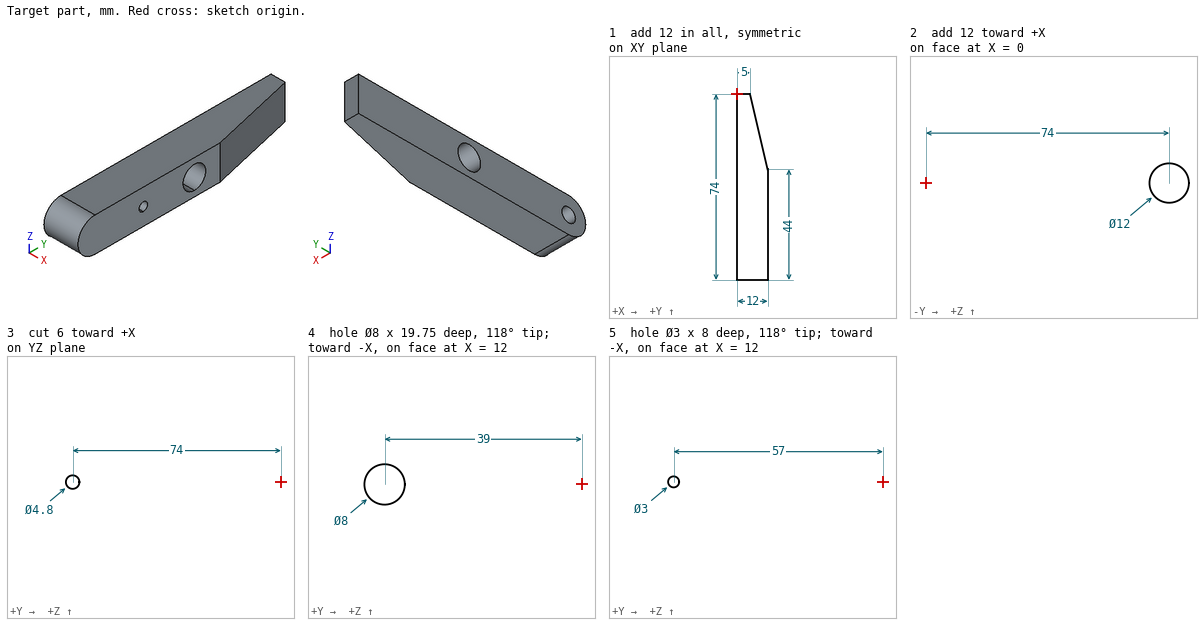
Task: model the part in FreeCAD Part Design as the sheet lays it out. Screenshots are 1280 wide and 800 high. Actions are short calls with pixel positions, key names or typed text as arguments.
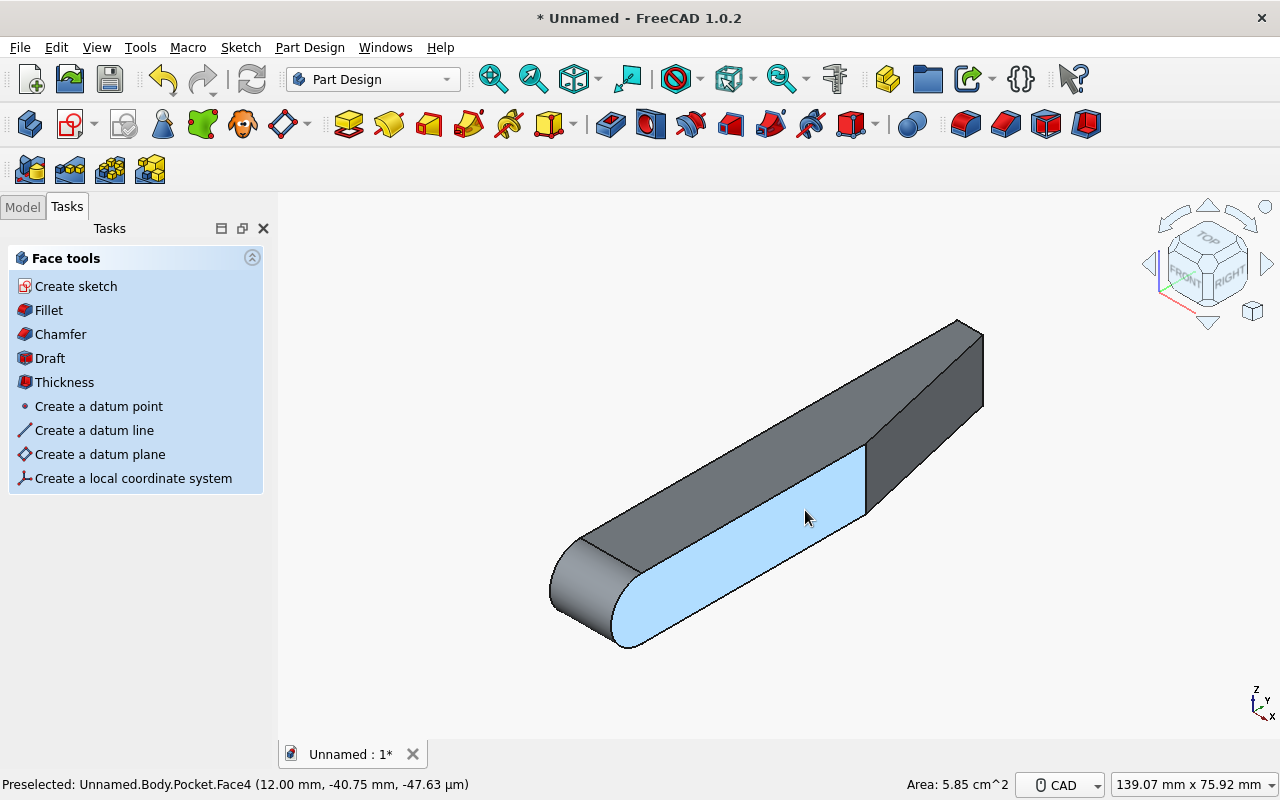
click(70, 124)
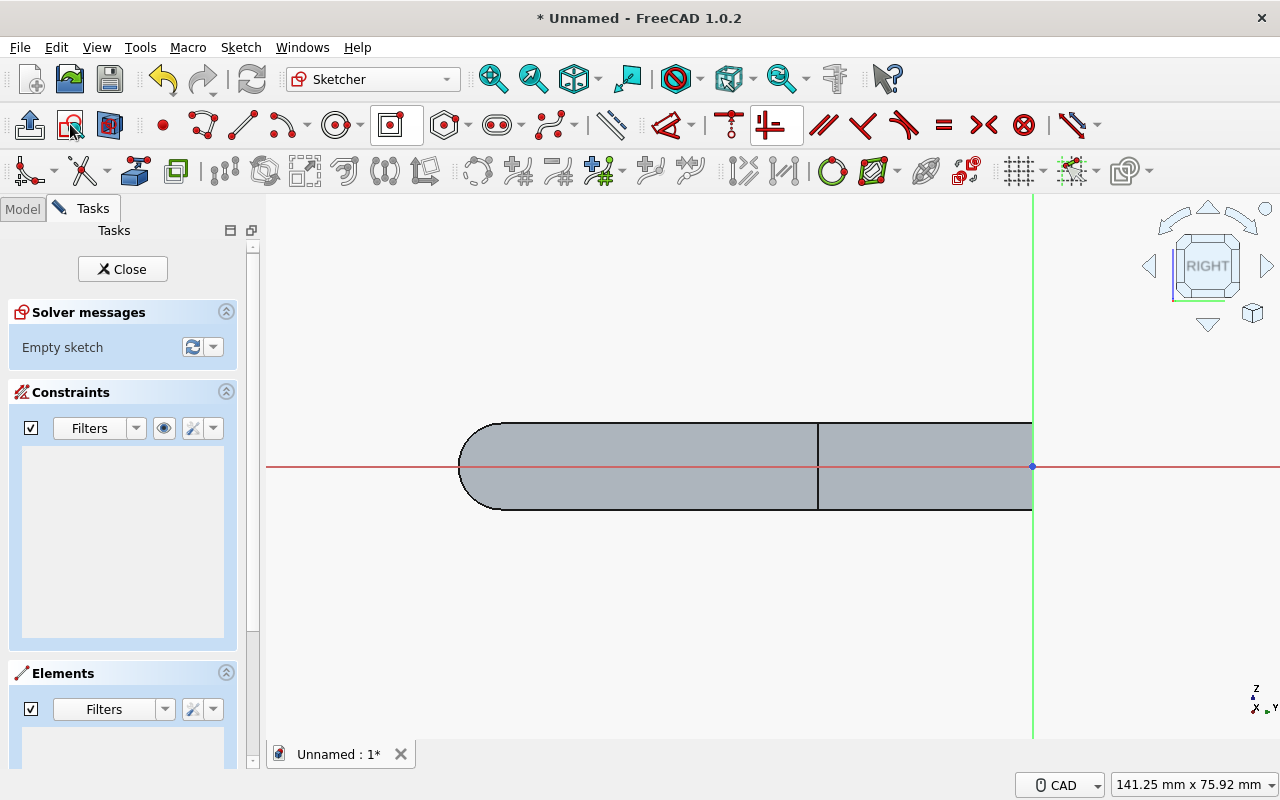
scroll(762, 467, up, 9)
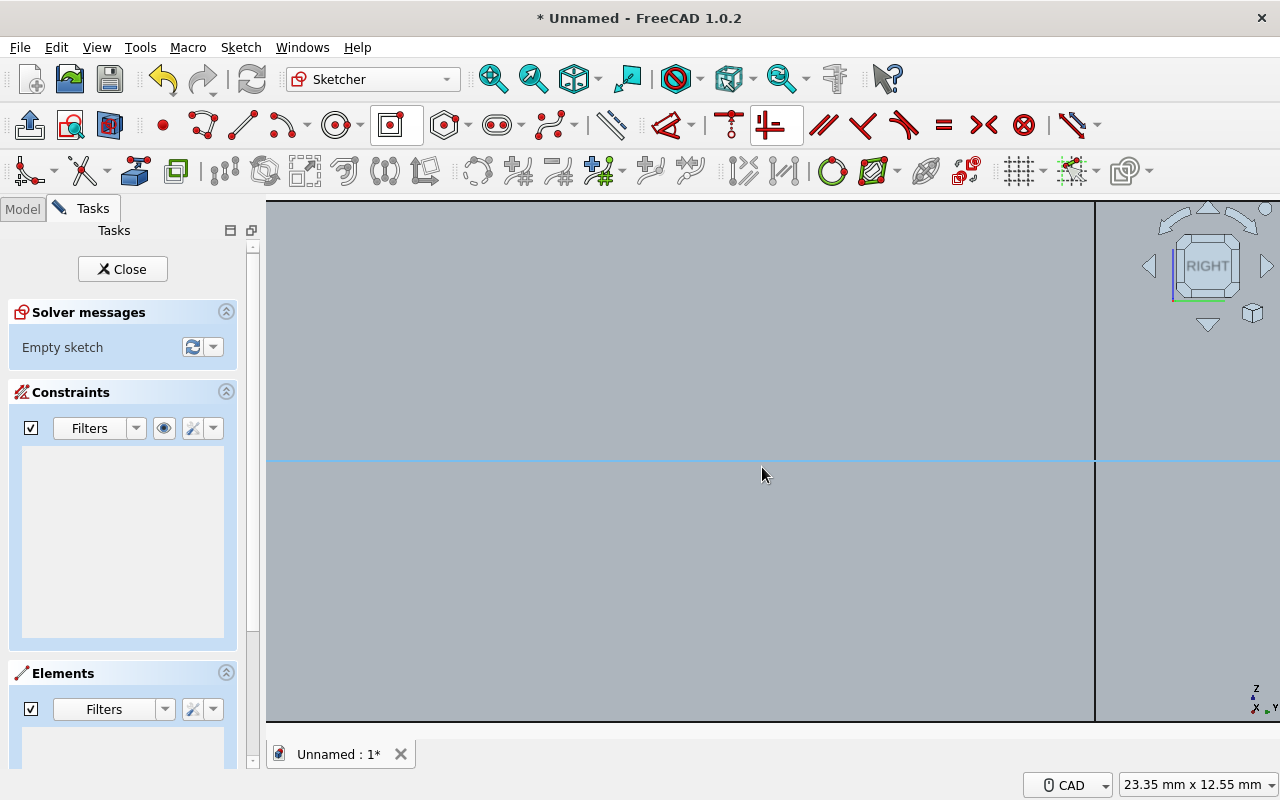
click(336, 126)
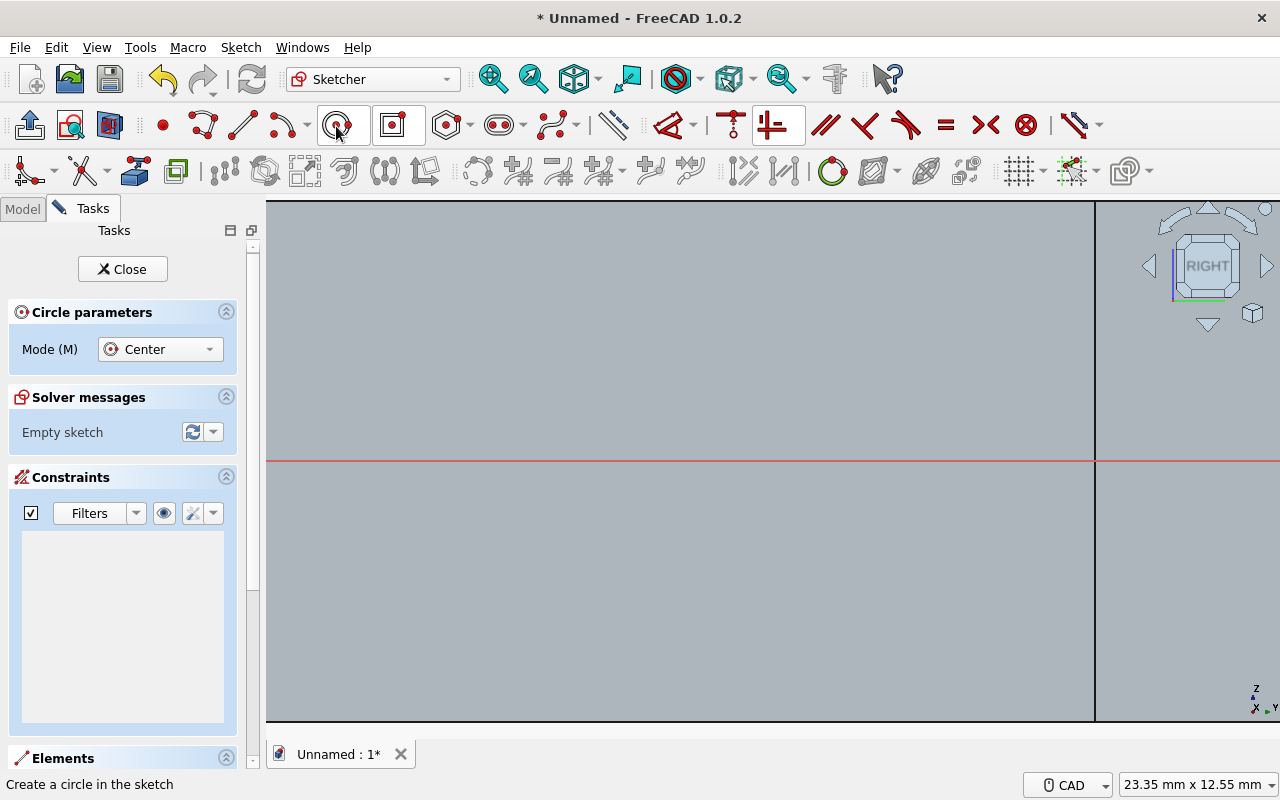
click(705, 461)
move(827, 339)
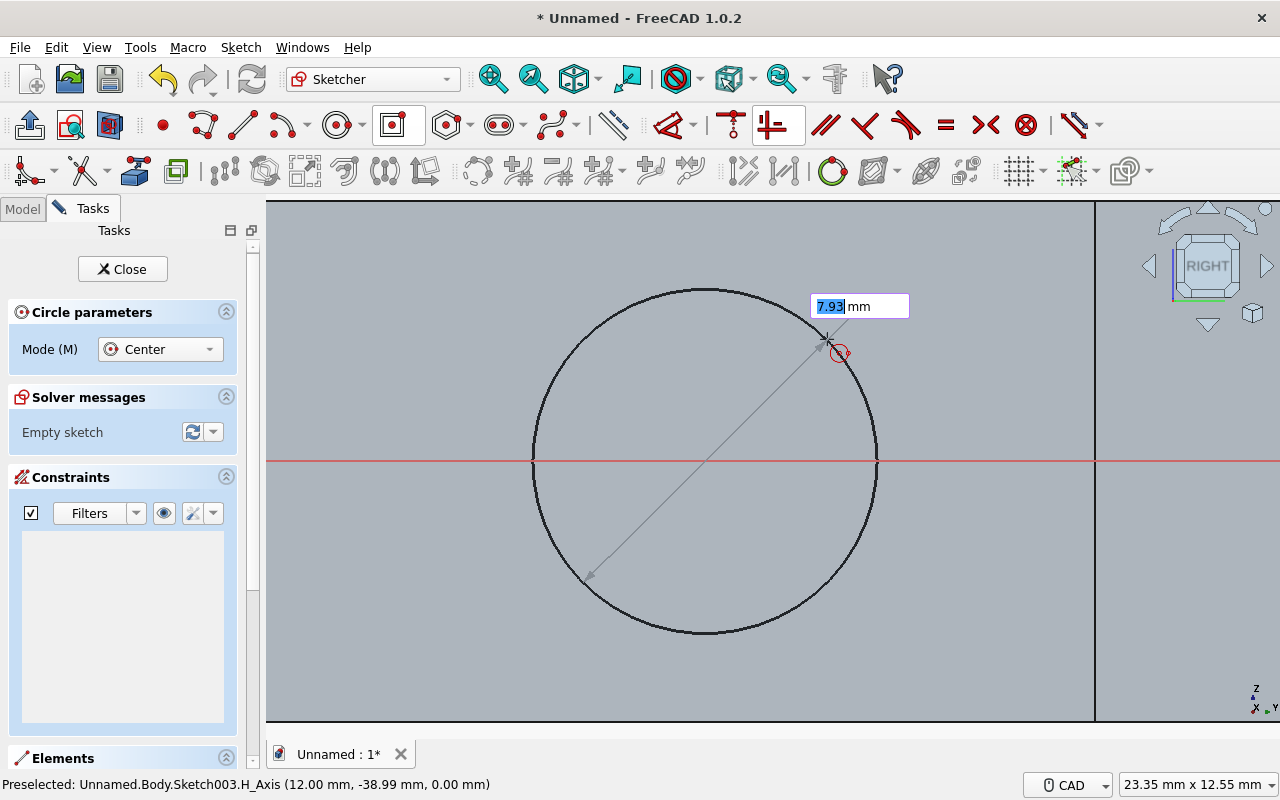
text(8)
key(Return)
key(Escape)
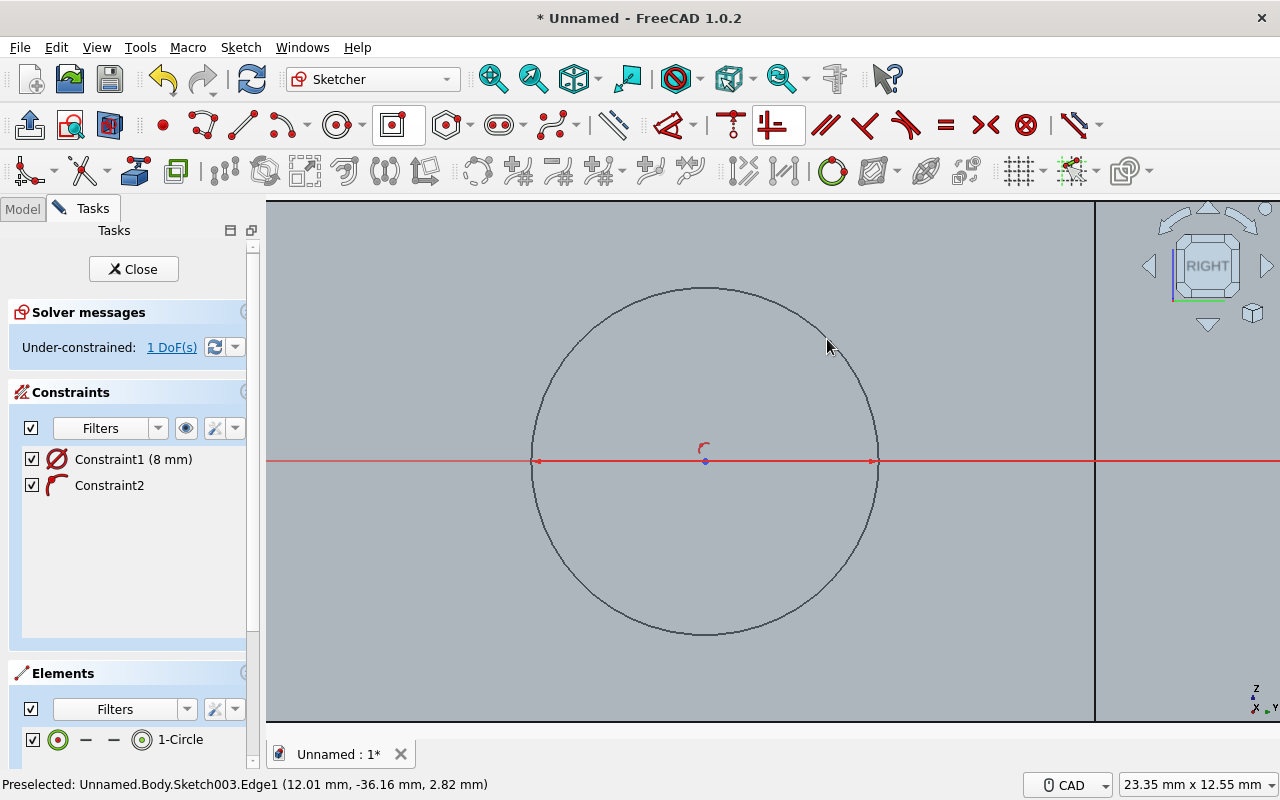
click(668, 126)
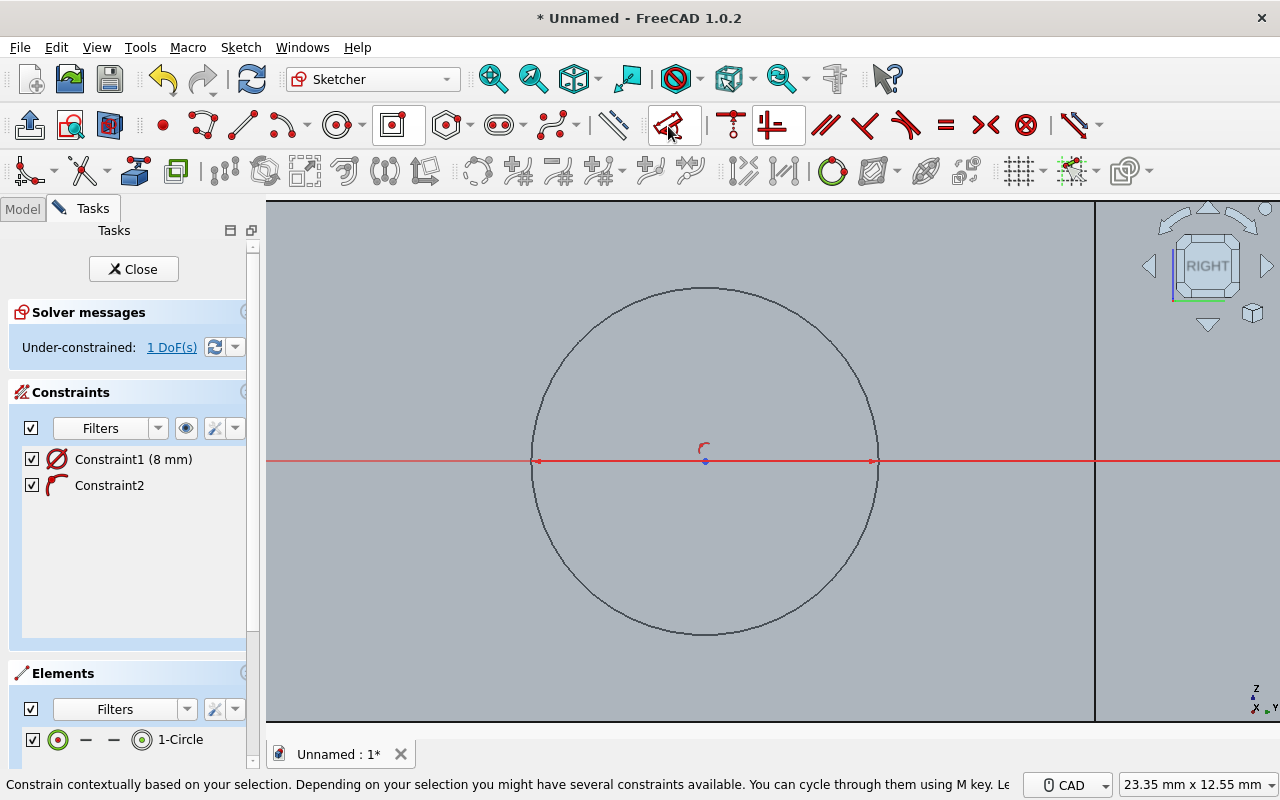
click(705, 461)
click(910, 495)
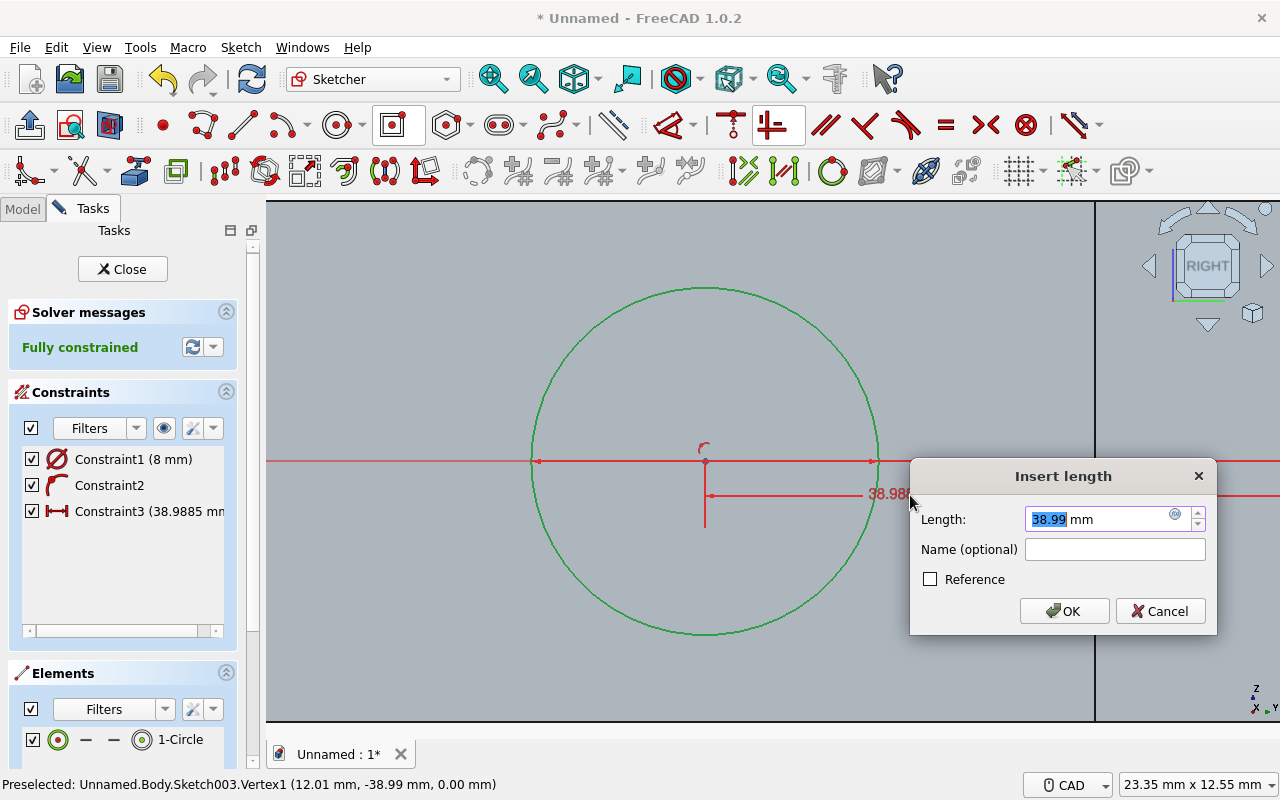
text(39)
key(Return)
key(Escape)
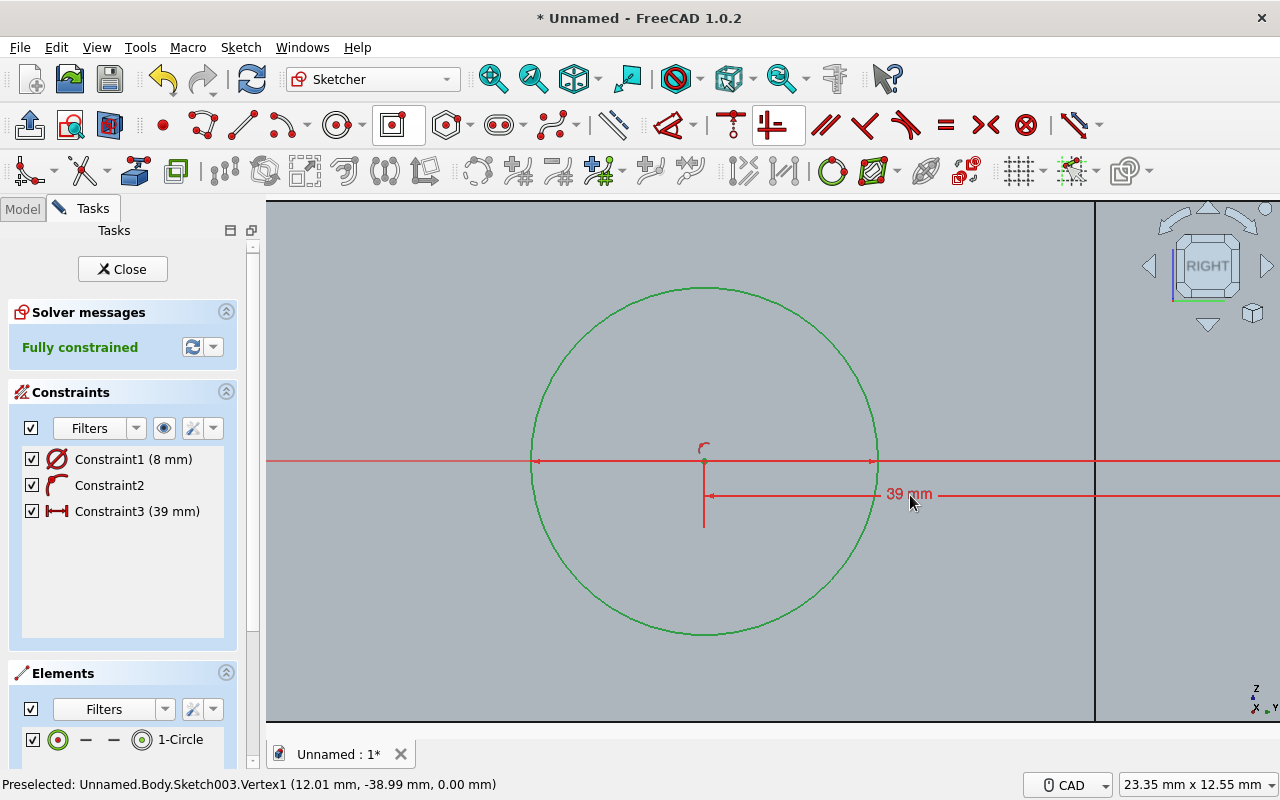
click(123, 269)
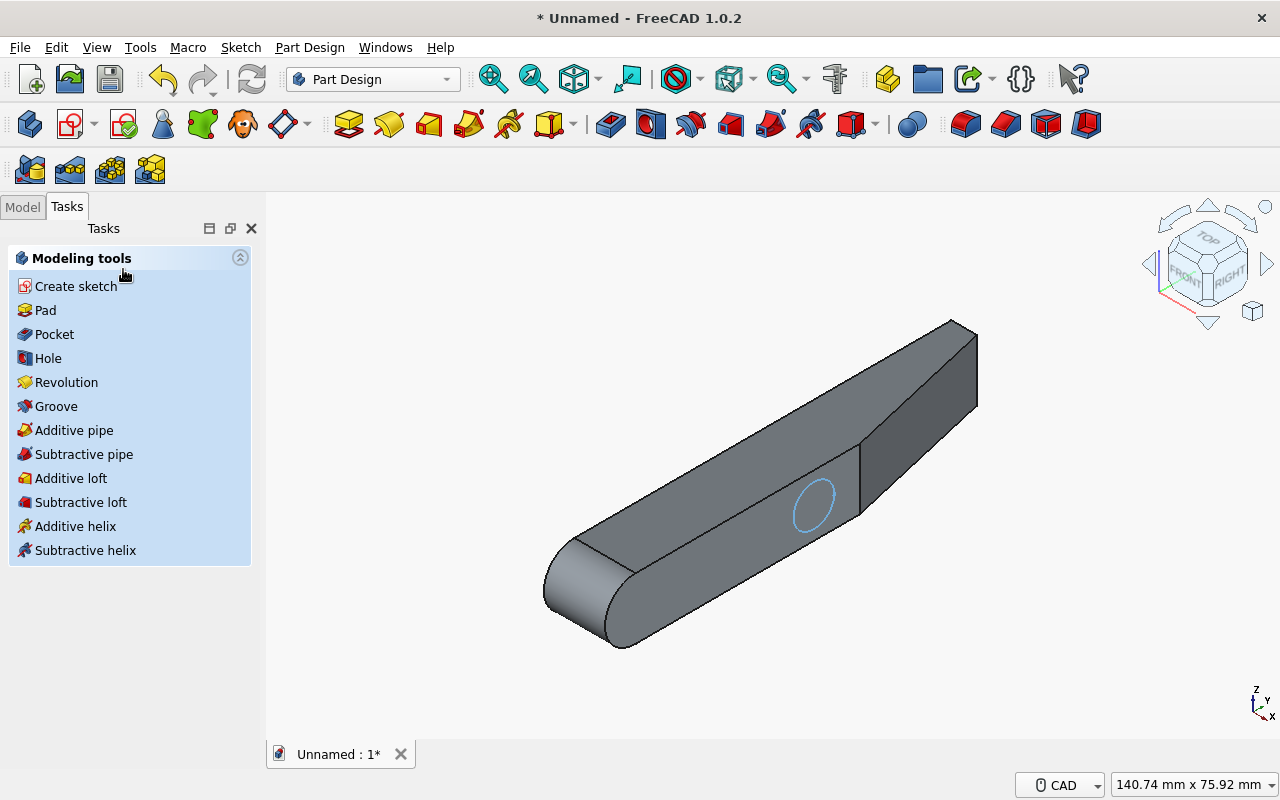
click(652, 124)